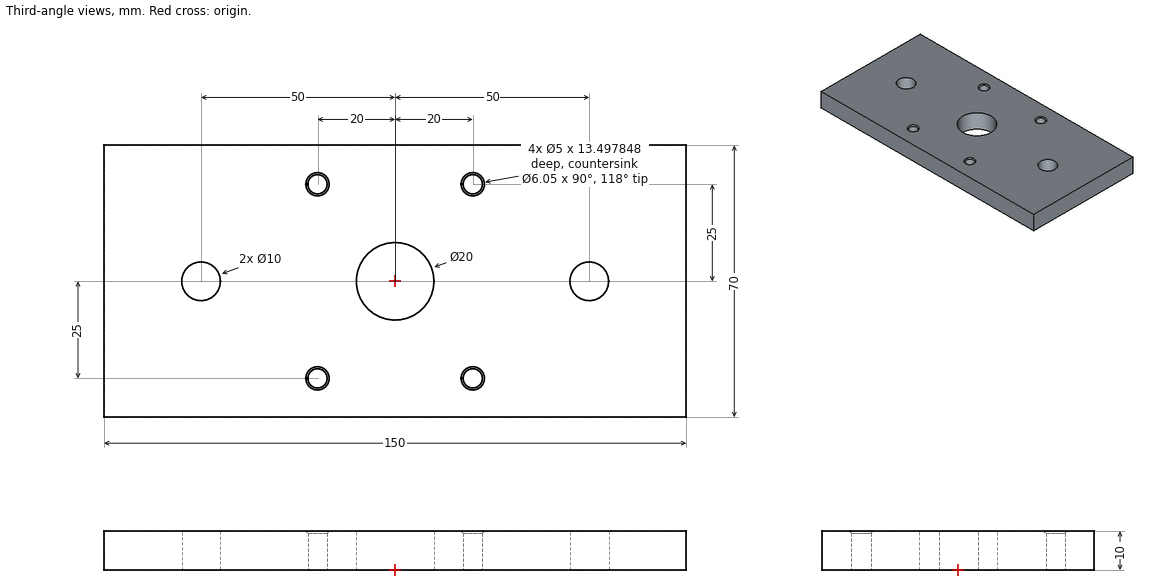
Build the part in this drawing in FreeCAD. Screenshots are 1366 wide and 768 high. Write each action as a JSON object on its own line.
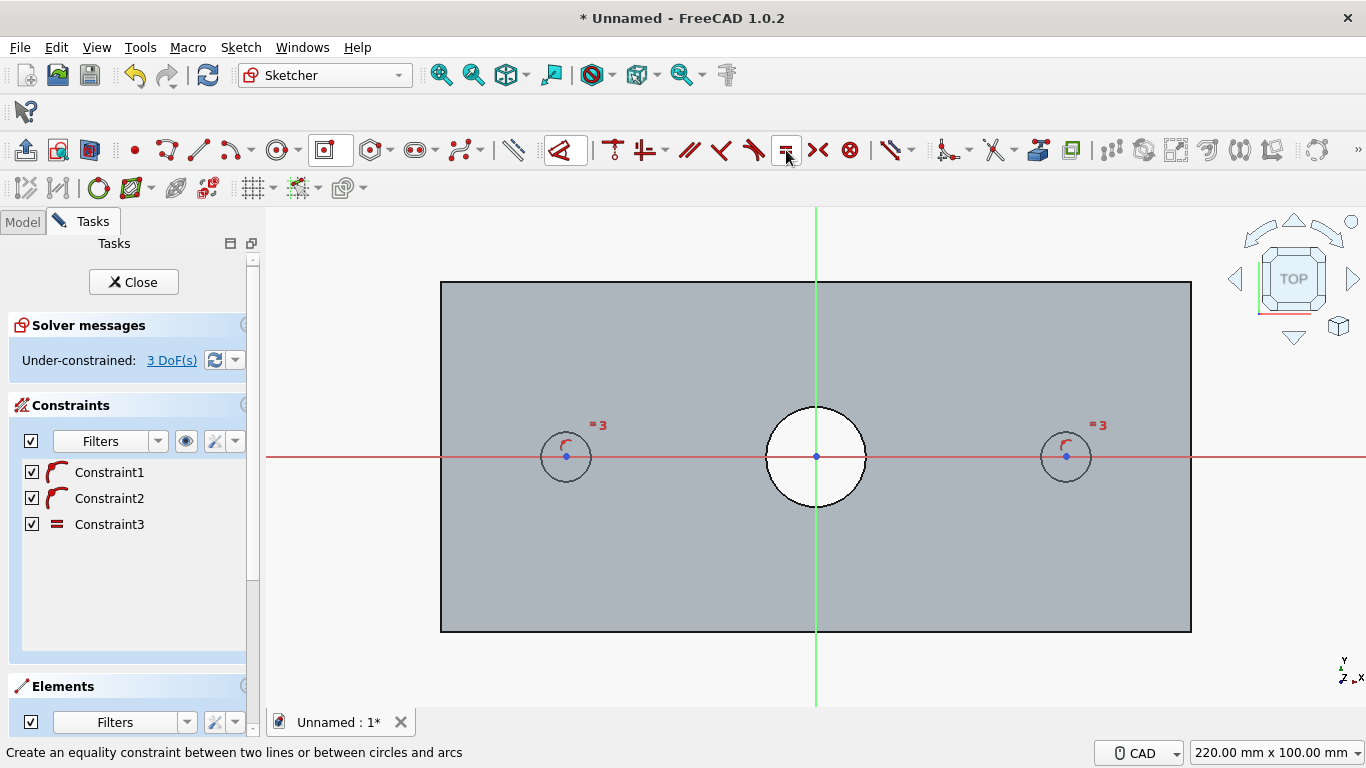
{"action": "left_click", "coordinate": [583, 439]}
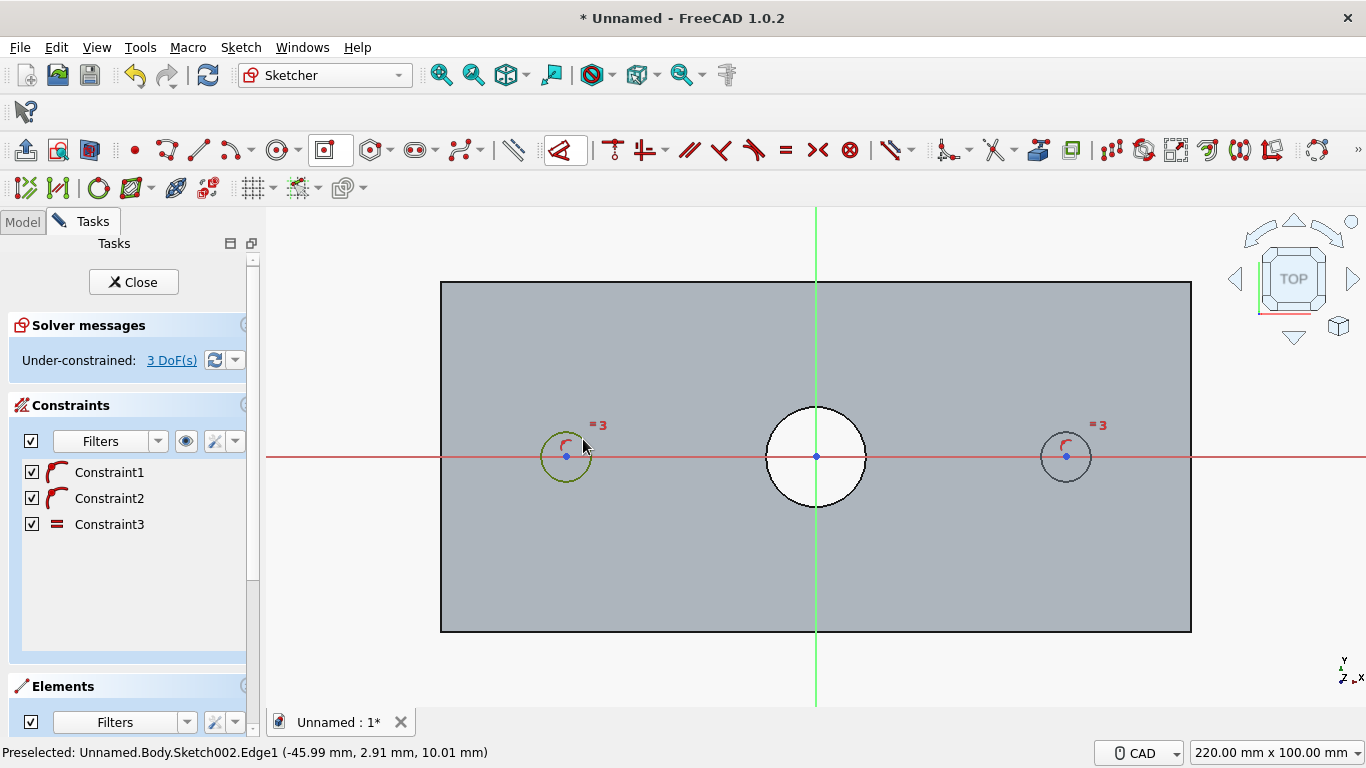
{"action": "left_click", "coordinate": [582, 150]}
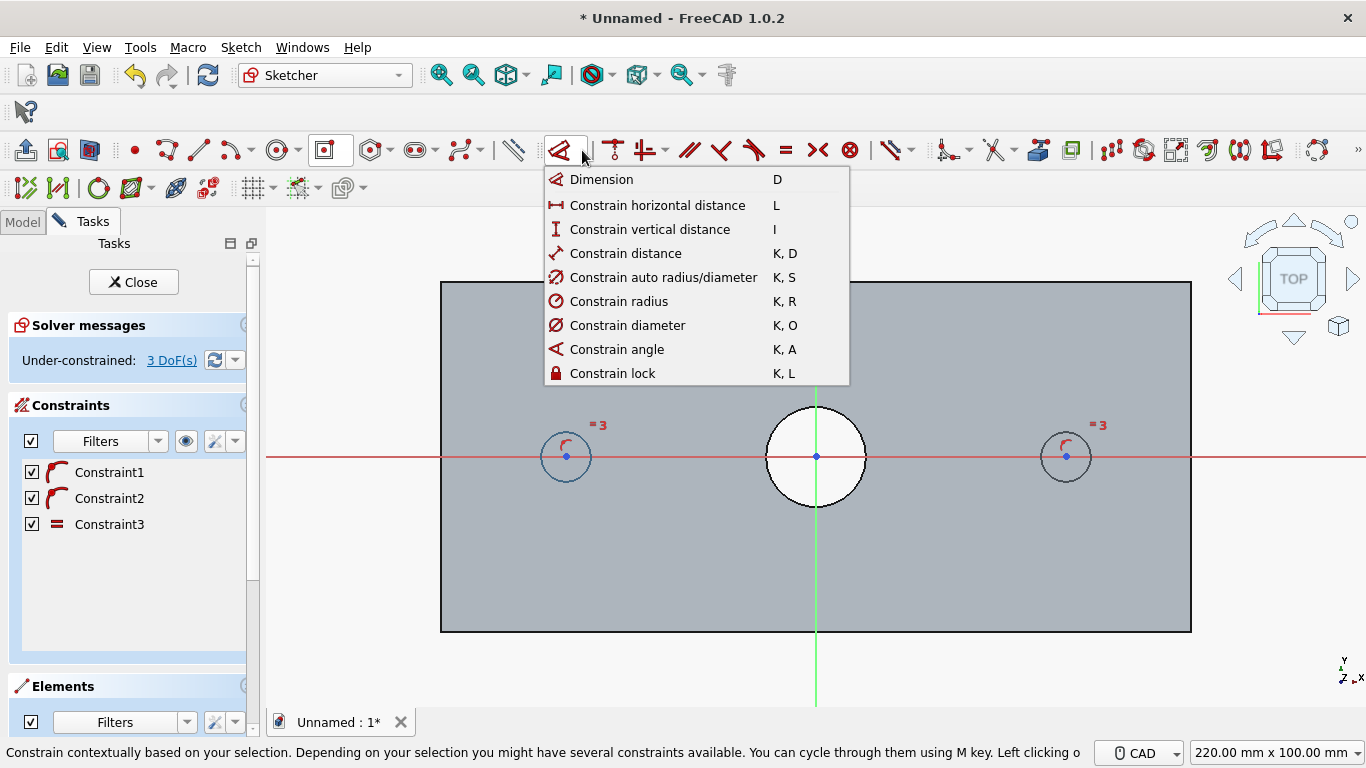
{"action": "left_click", "coordinate": [697, 325]}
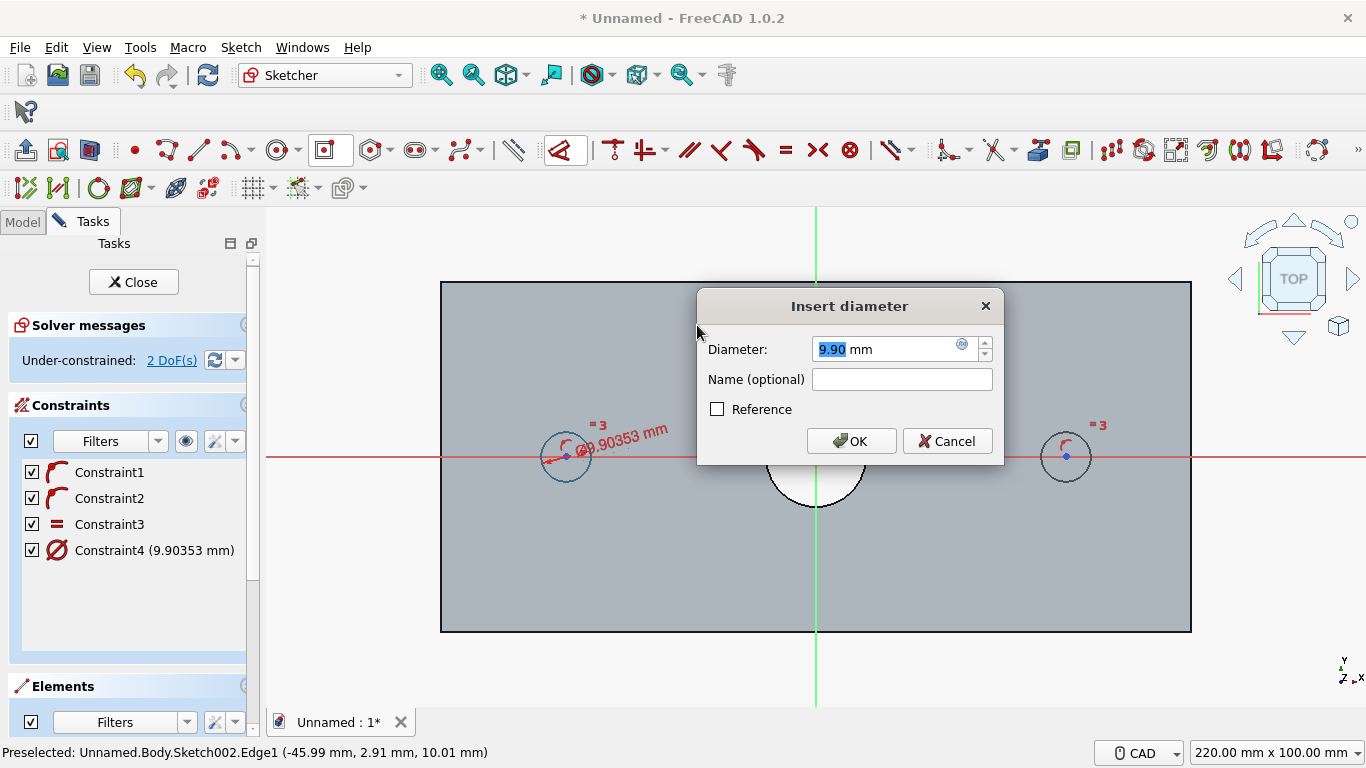
{"action": "type", "text": "10"}
{"action": "key", "text": "Return"}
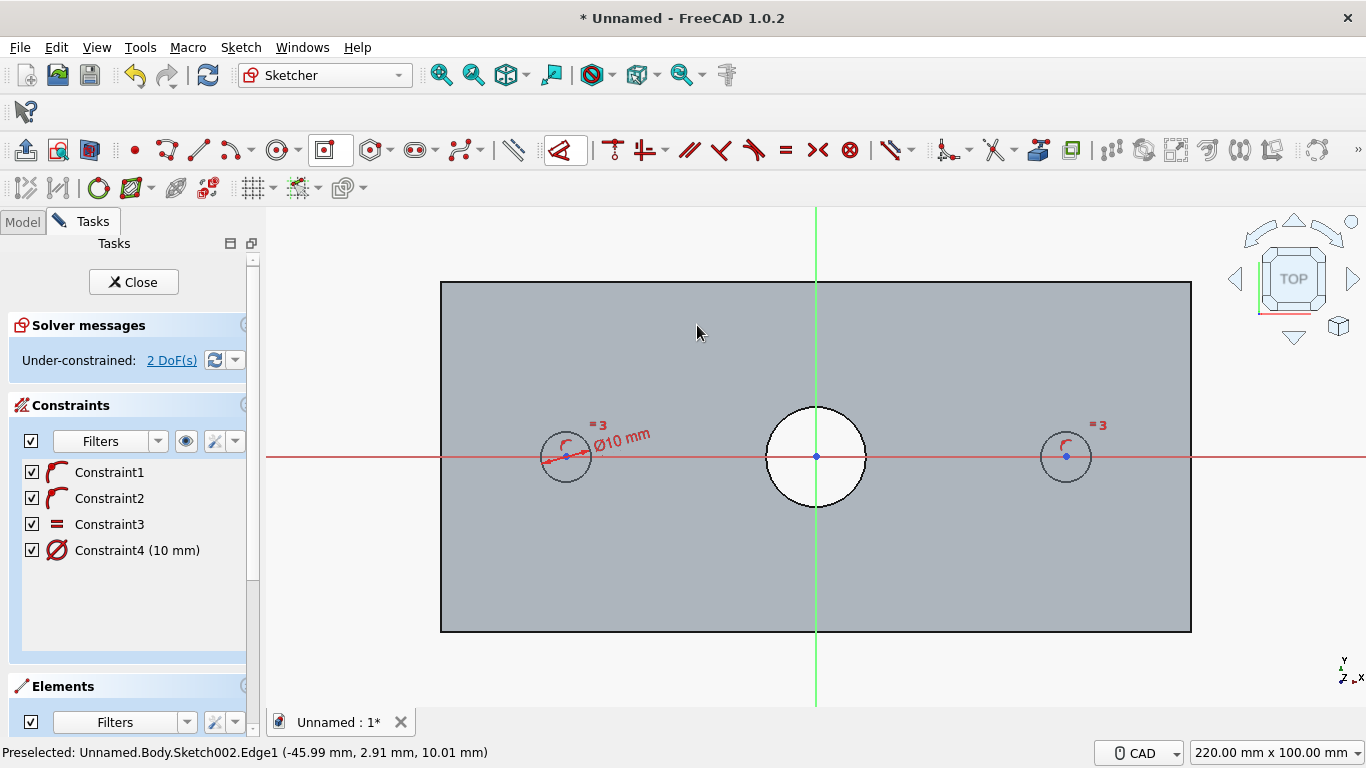
{"action": "left_click", "coordinate": [566, 457]}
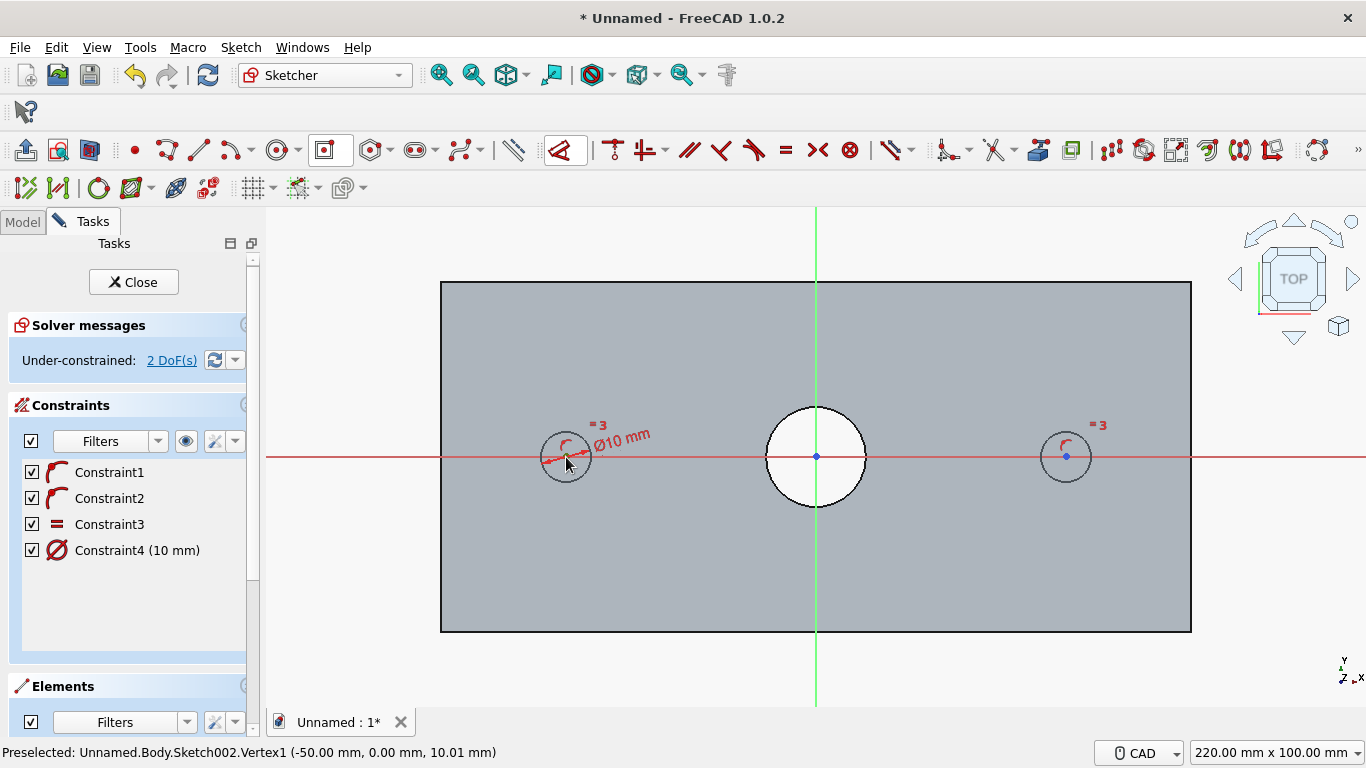
{"action": "key", "text": "l"}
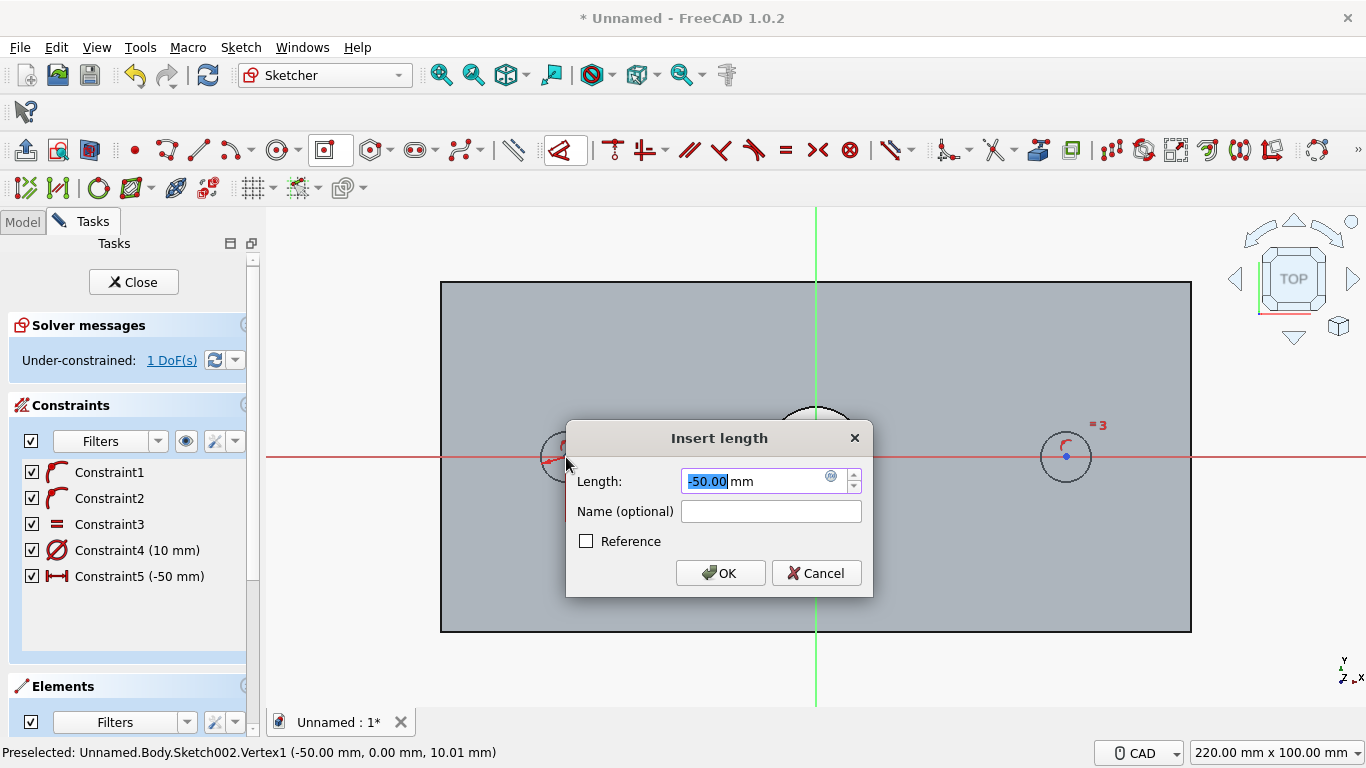
{"action": "type", "text": "-50"}
{"action": "key", "text": "Return"}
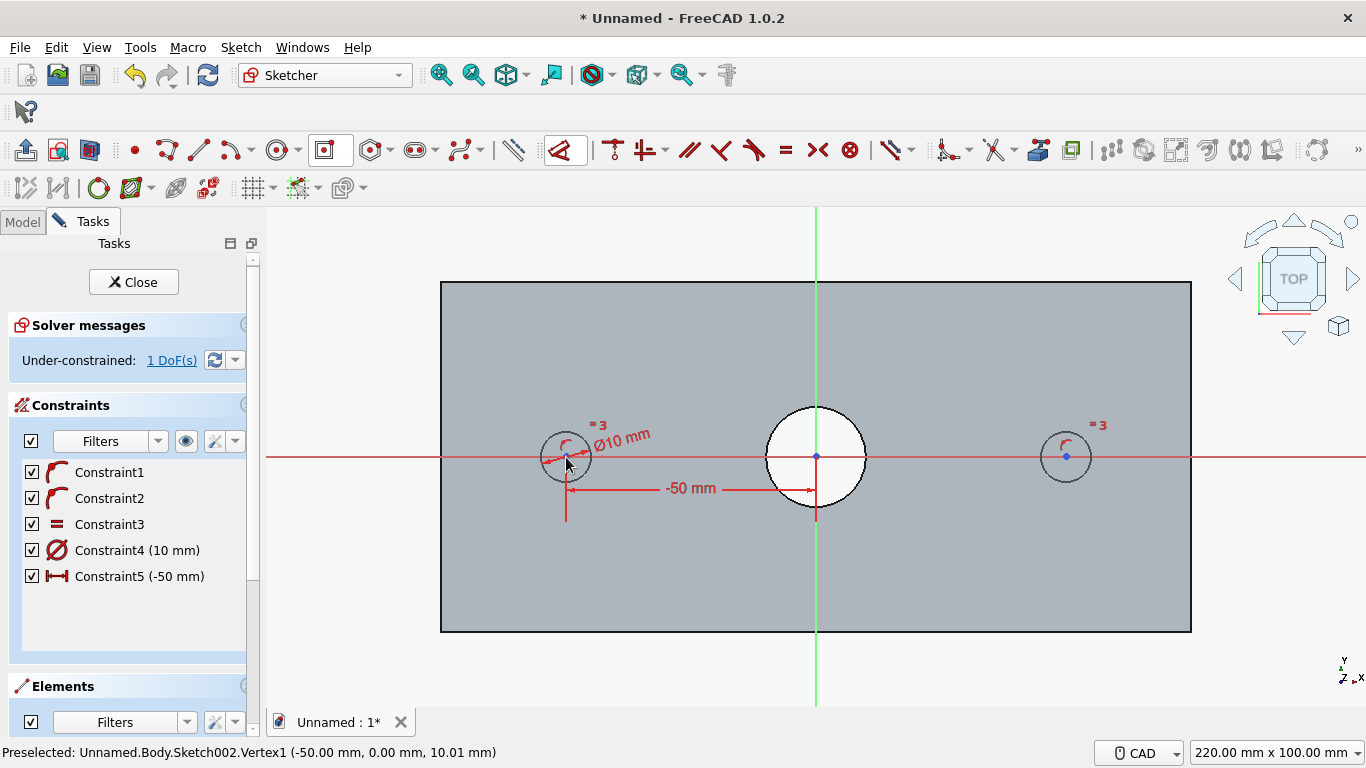
{"action": "left_click", "coordinate": [1066, 457]}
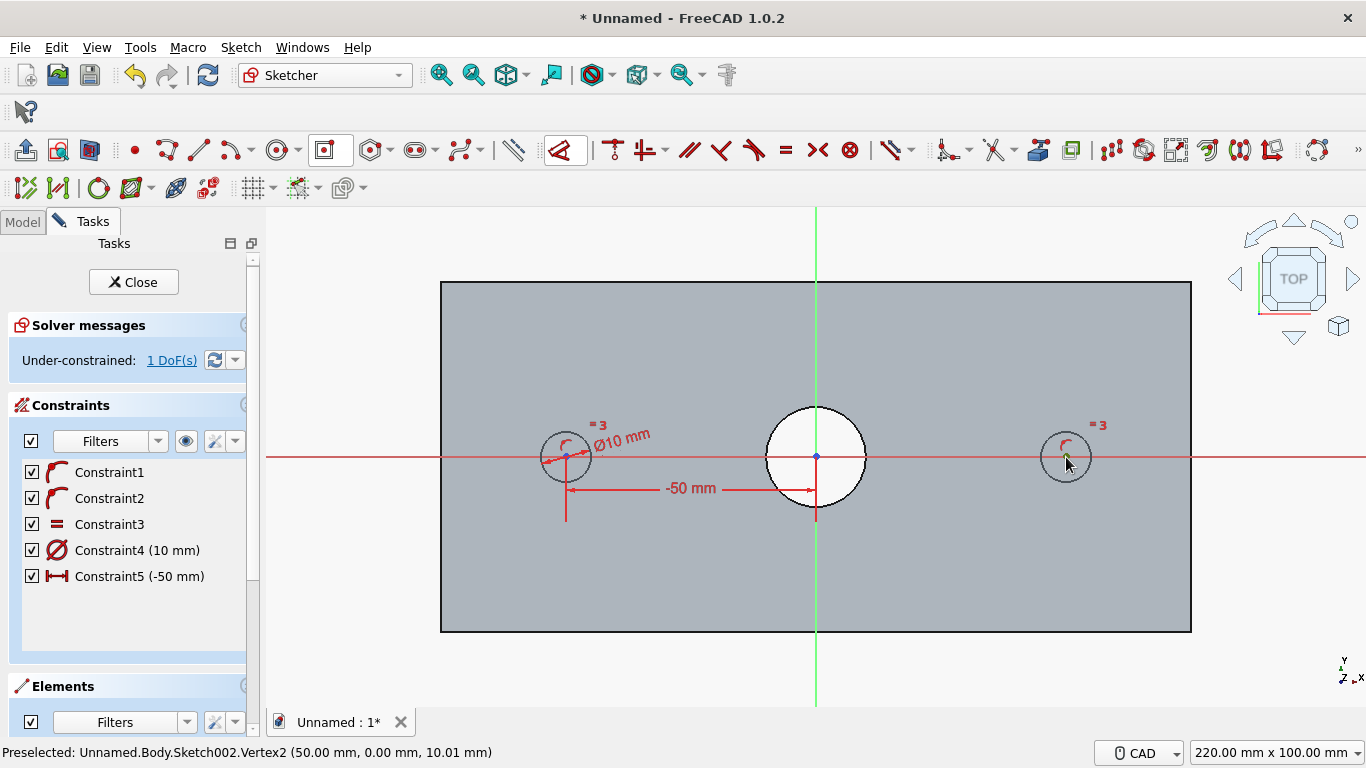
{"action": "left_click", "coordinate": [582, 150]}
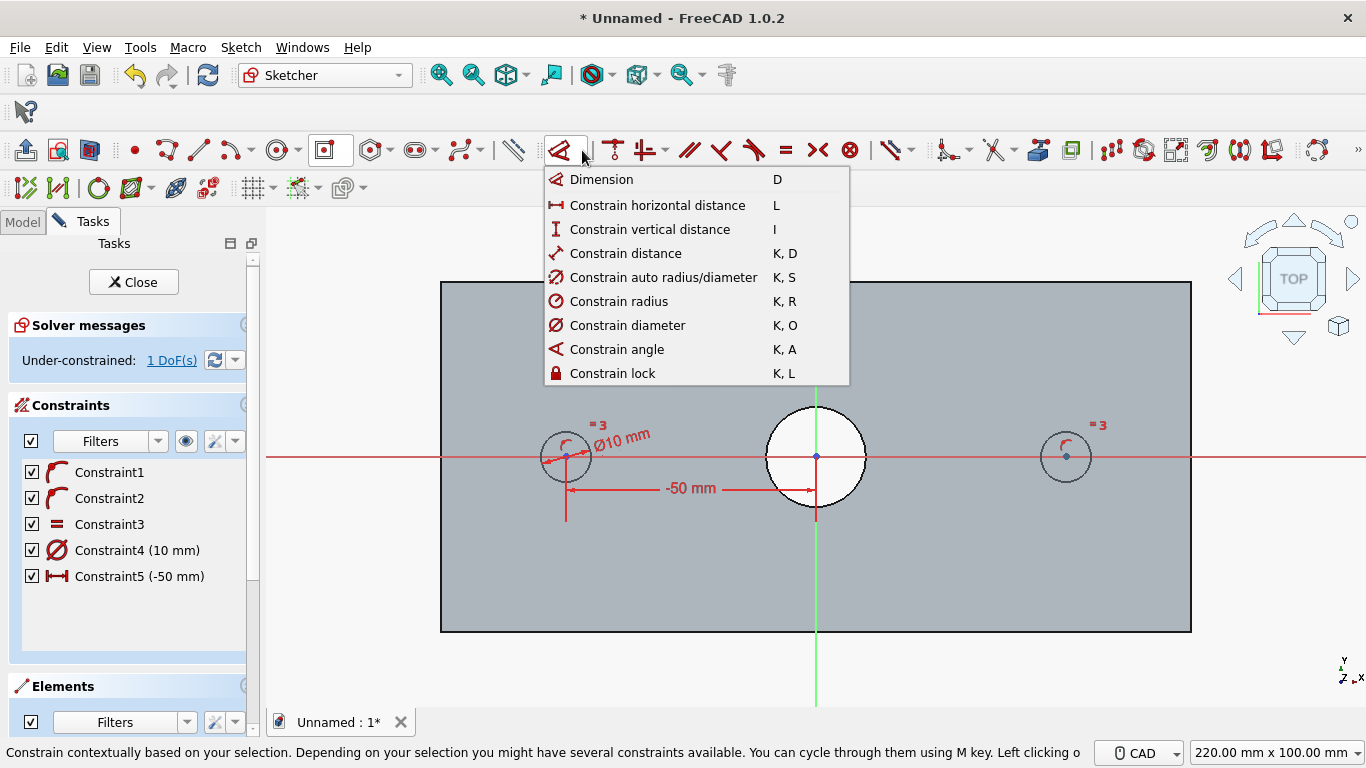
{"action": "left_click", "coordinate": [697, 205]}